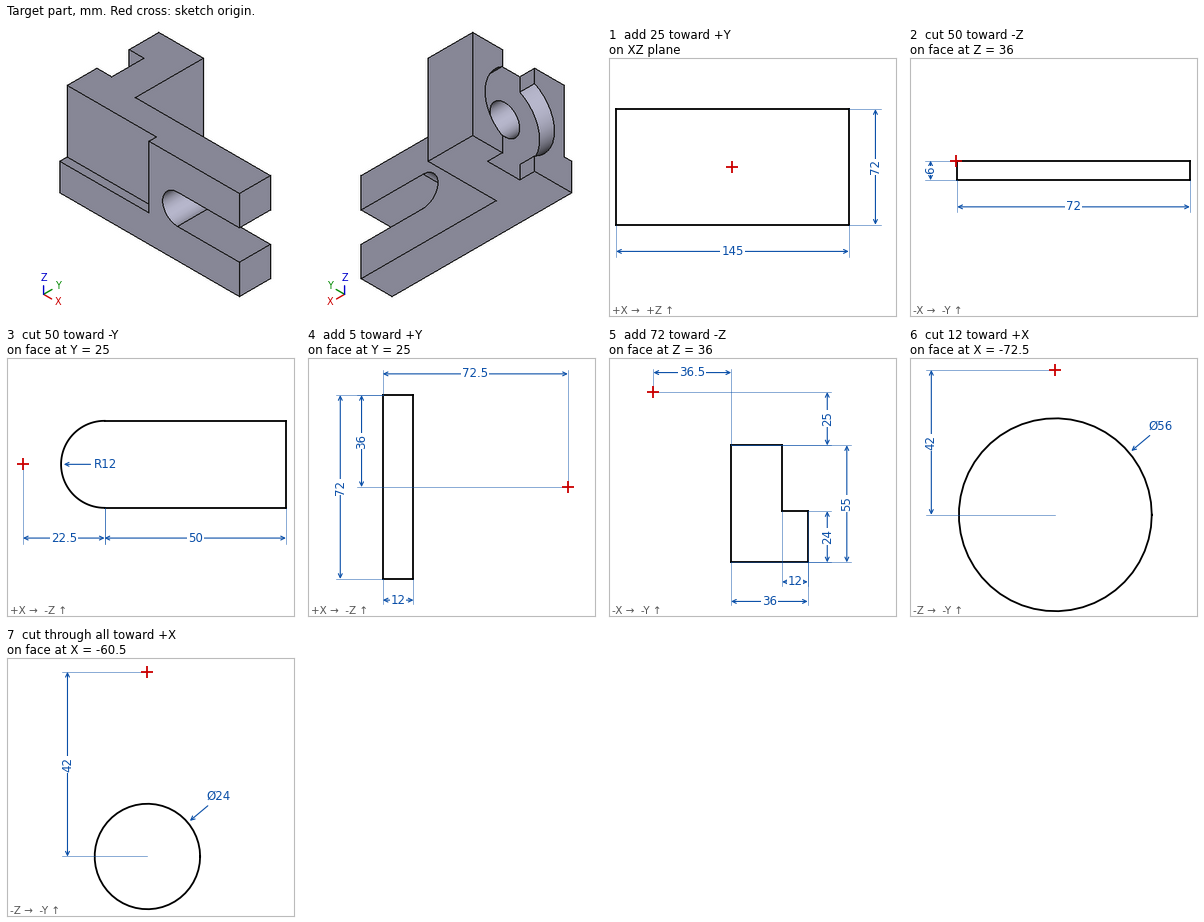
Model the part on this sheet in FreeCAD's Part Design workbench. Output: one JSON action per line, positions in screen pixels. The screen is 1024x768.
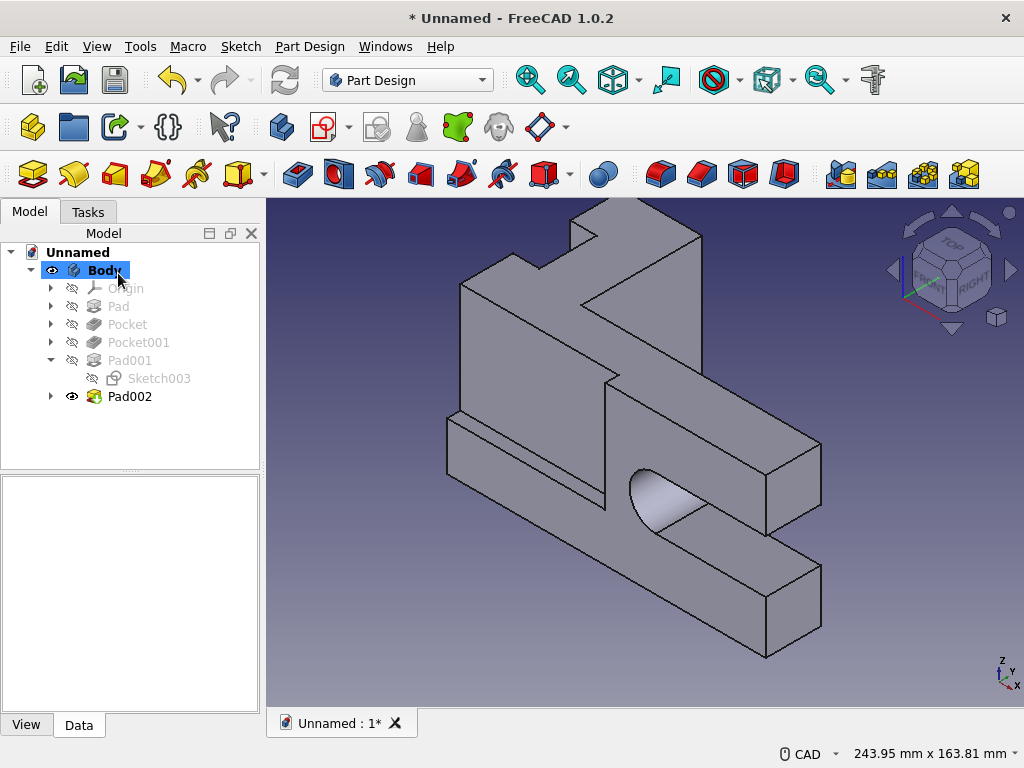
{"action": "left_click", "coordinate": [531, 80]}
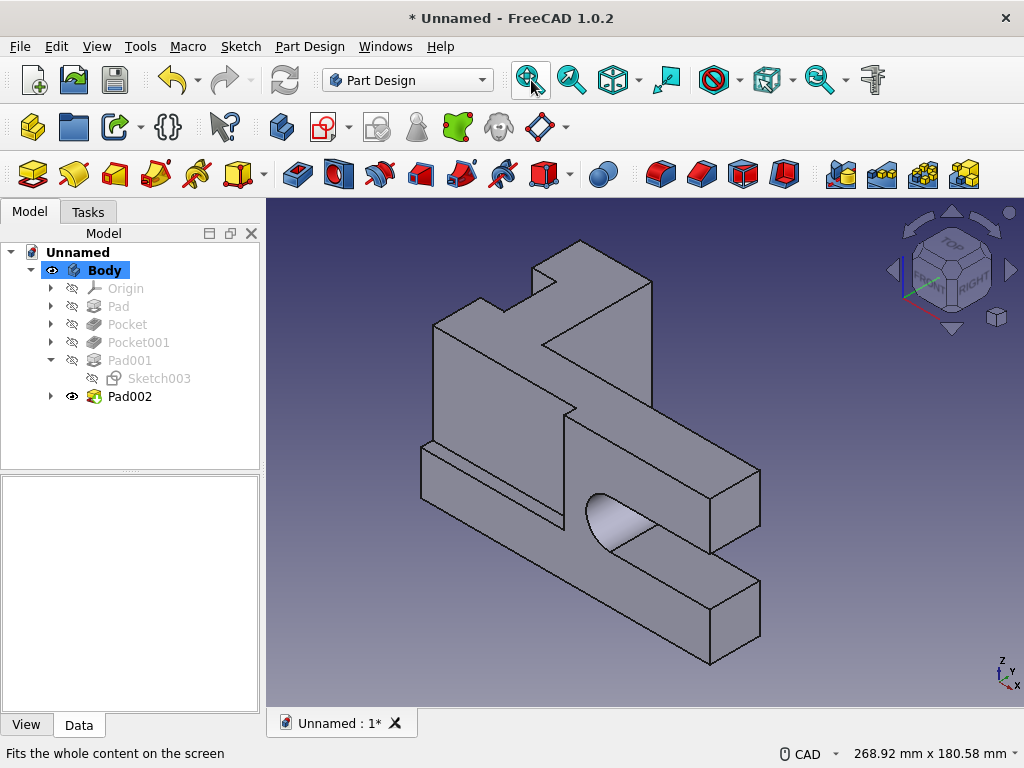
{"action": "key", "text": "6"}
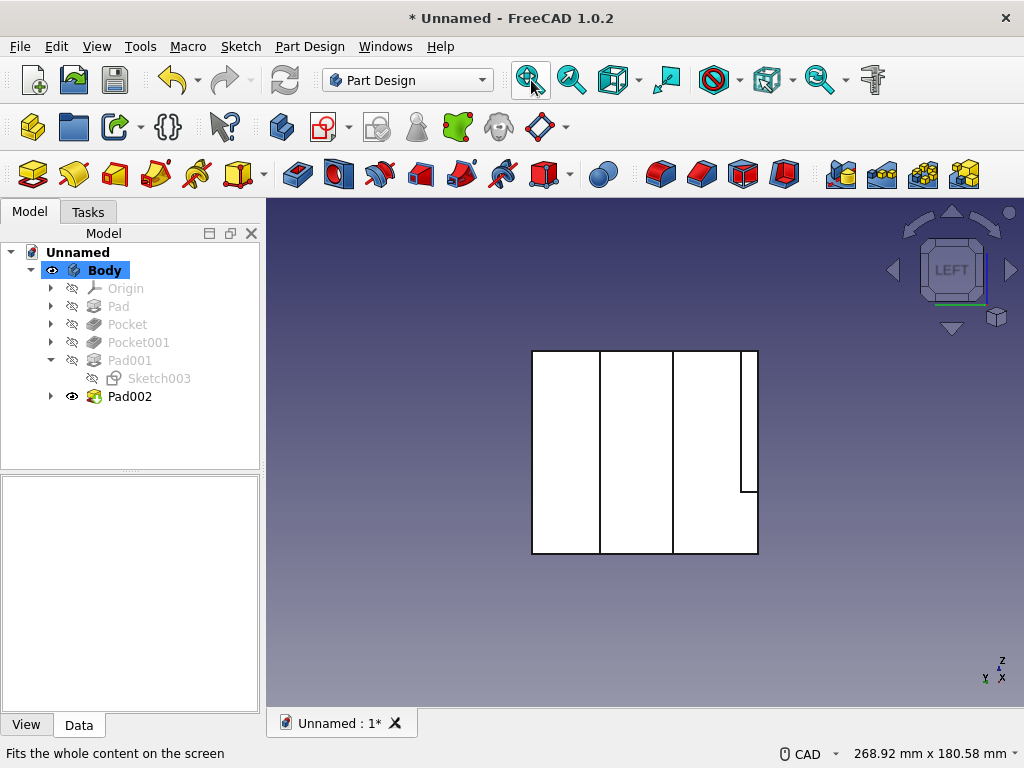
{"action": "left_click", "coordinate": [531, 80]}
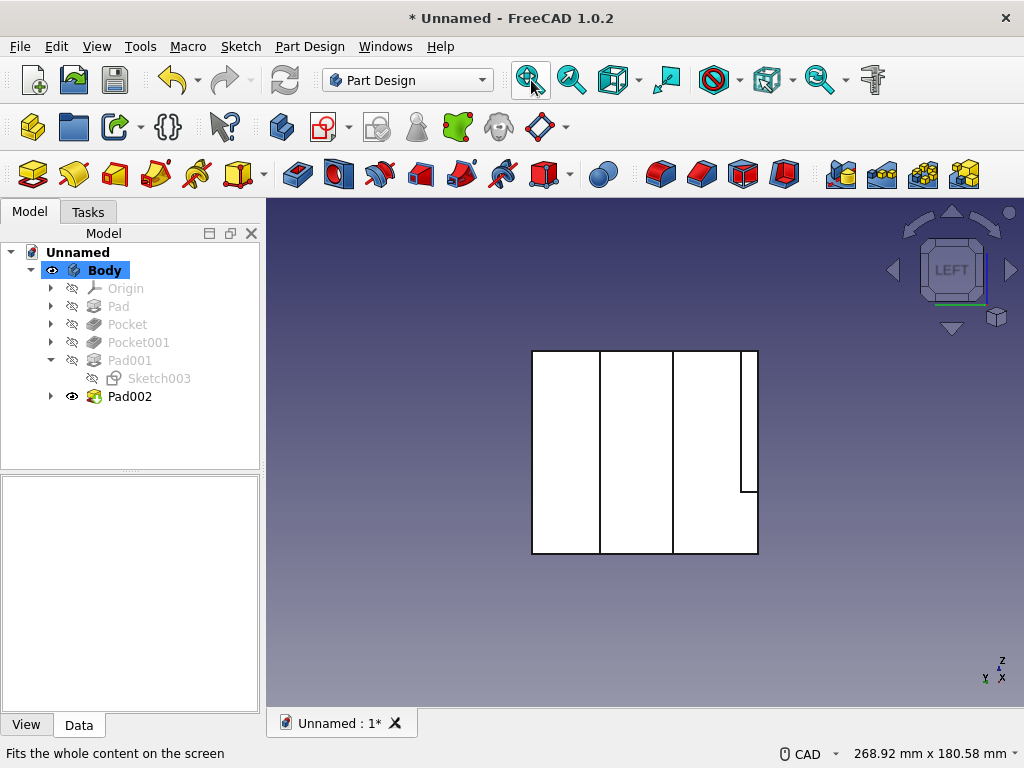
{"action": "left_click", "coordinate": [715, 509]}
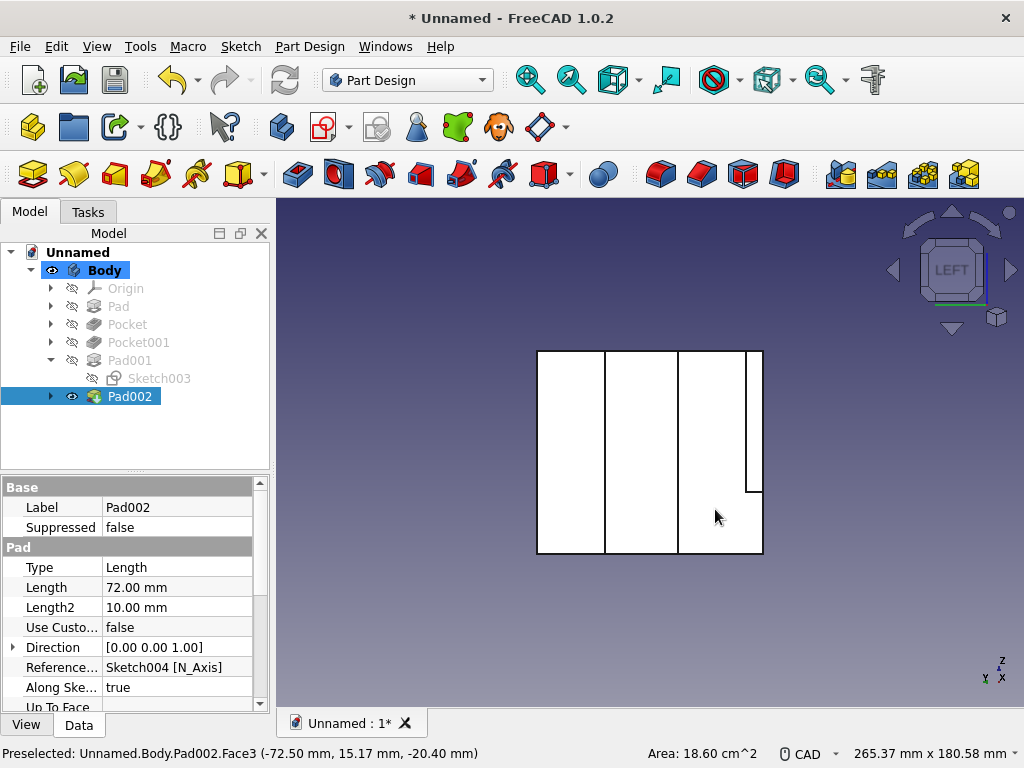
{"action": "left_click", "coordinate": [322, 128]}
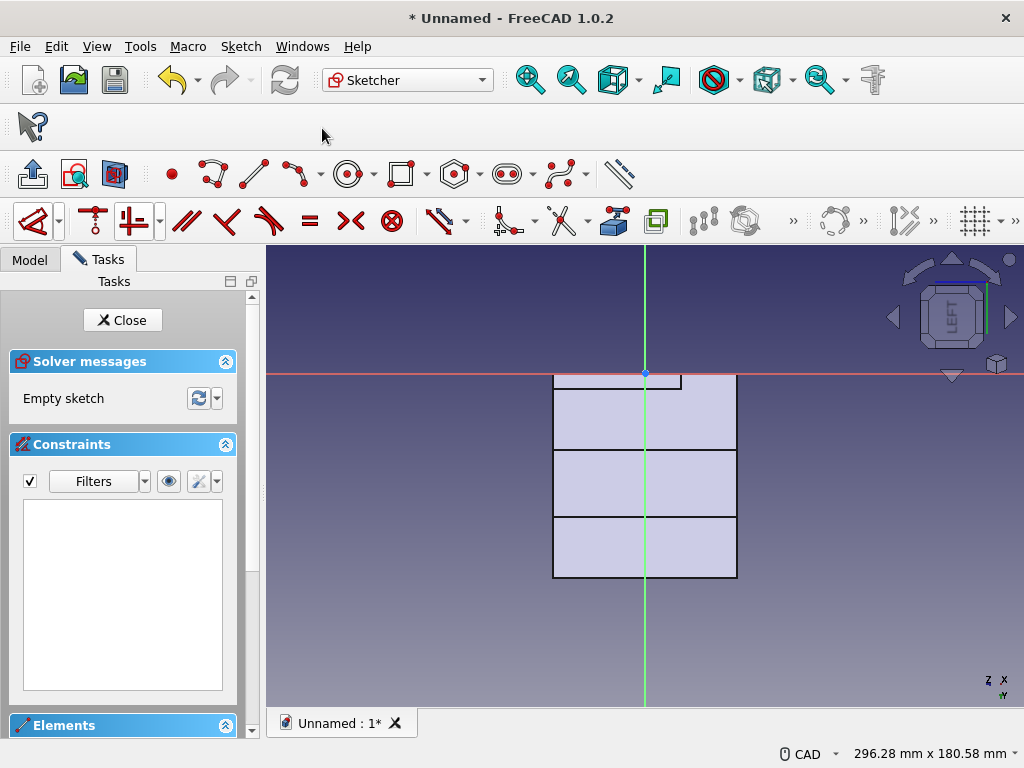
{"action": "scroll", "coordinate": [784, 437], "scroll_direction": "up", "scroll_amount": 2}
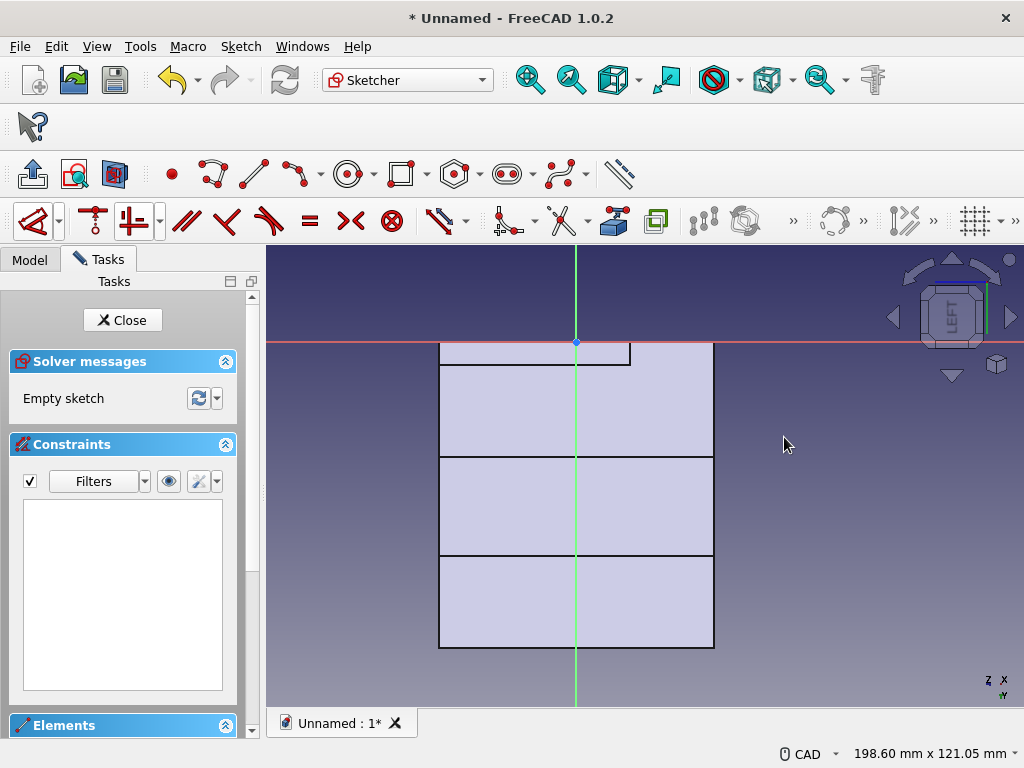
{"action": "left_click", "coordinate": [348, 174]}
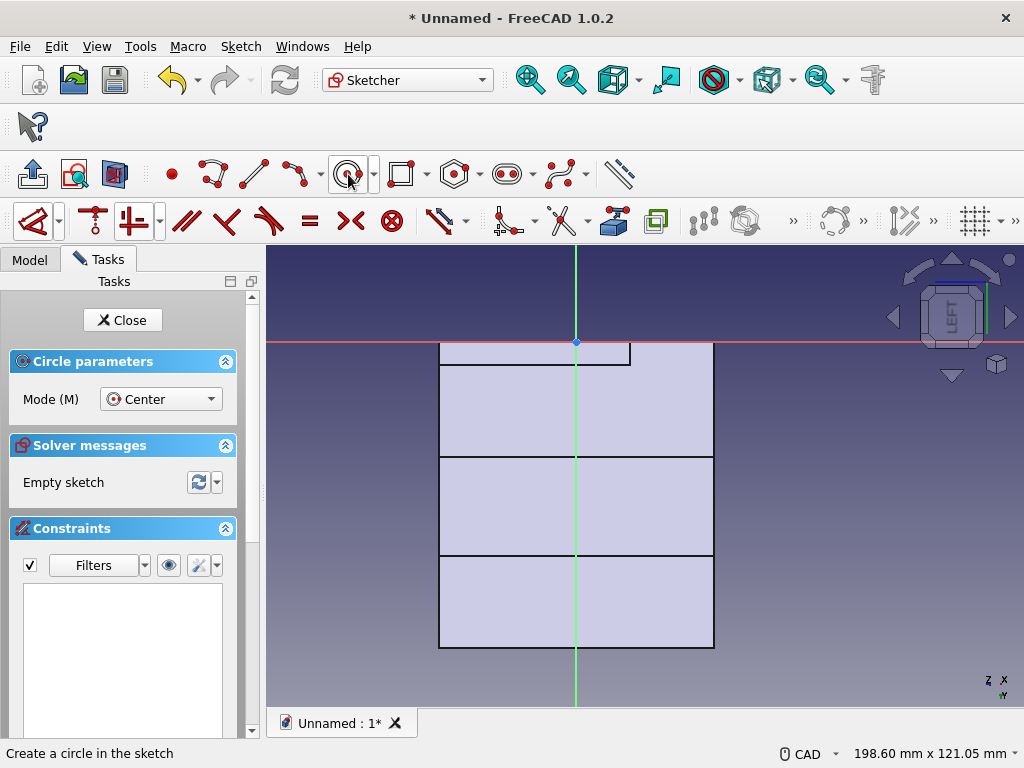
{"action": "left_click", "coordinate": [576, 503]}
{"action": "left_click", "coordinate": [652, 427]}
{"action": "key", "text": "Escape"}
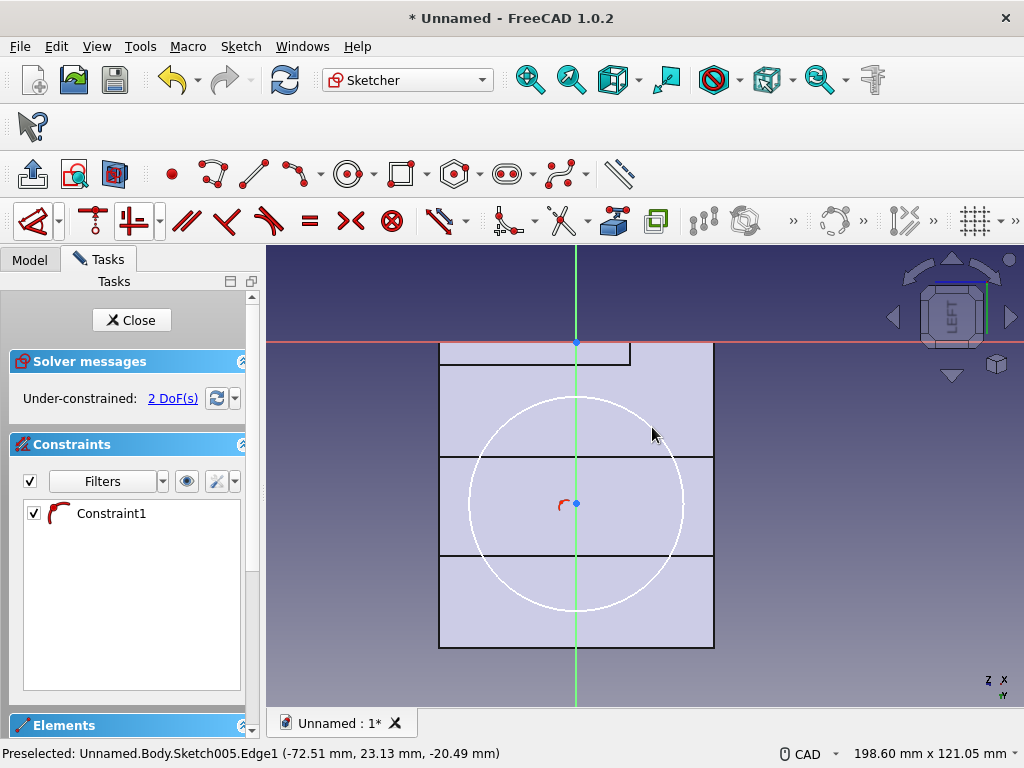
{"action": "left_click", "coordinate": [652, 428]}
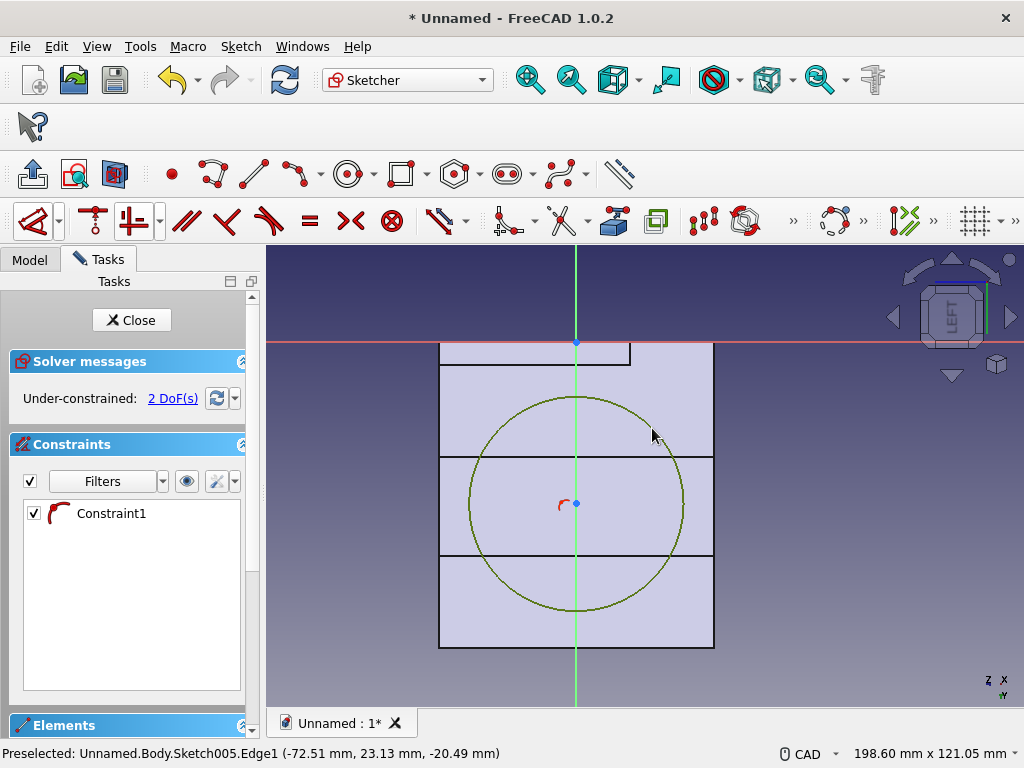
{"action": "key", "text": "k o"}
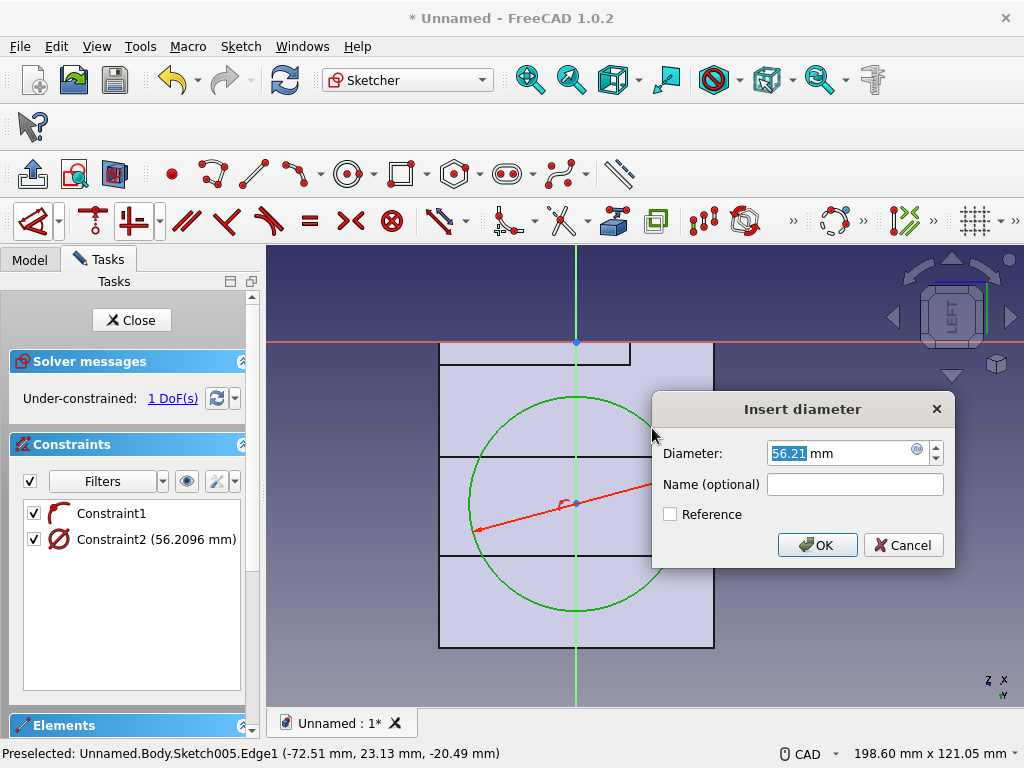
{"action": "type", "text": "56"}
{"action": "key", "text": "Return"}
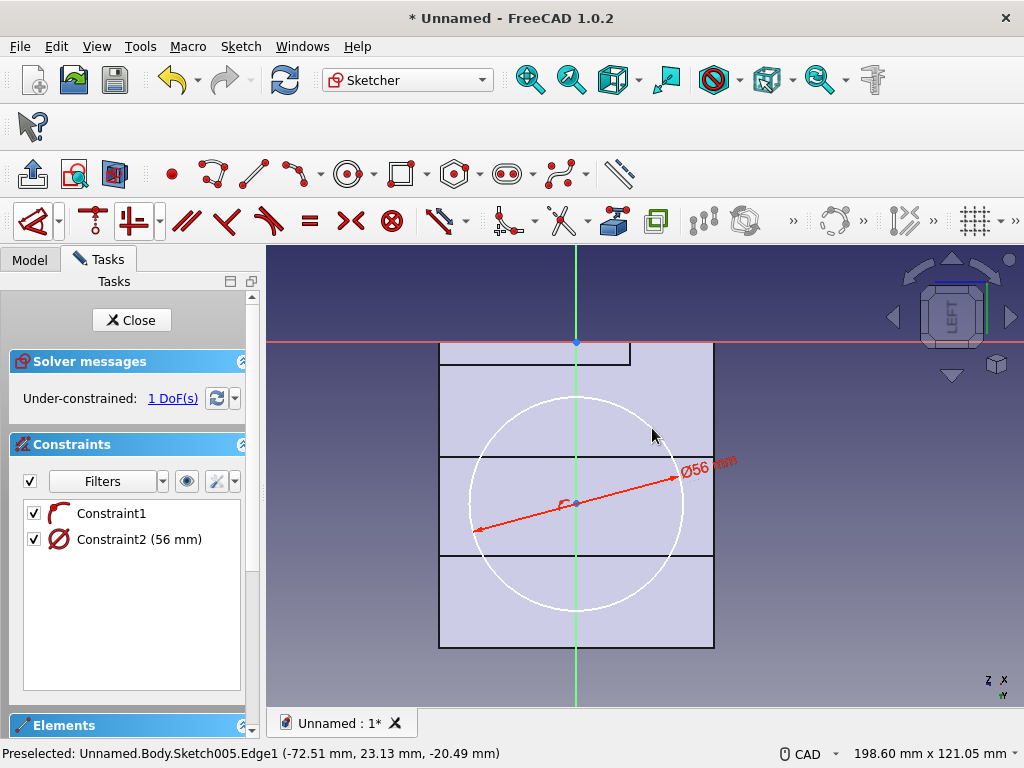
{"action": "left_click", "coordinate": [576, 504]}